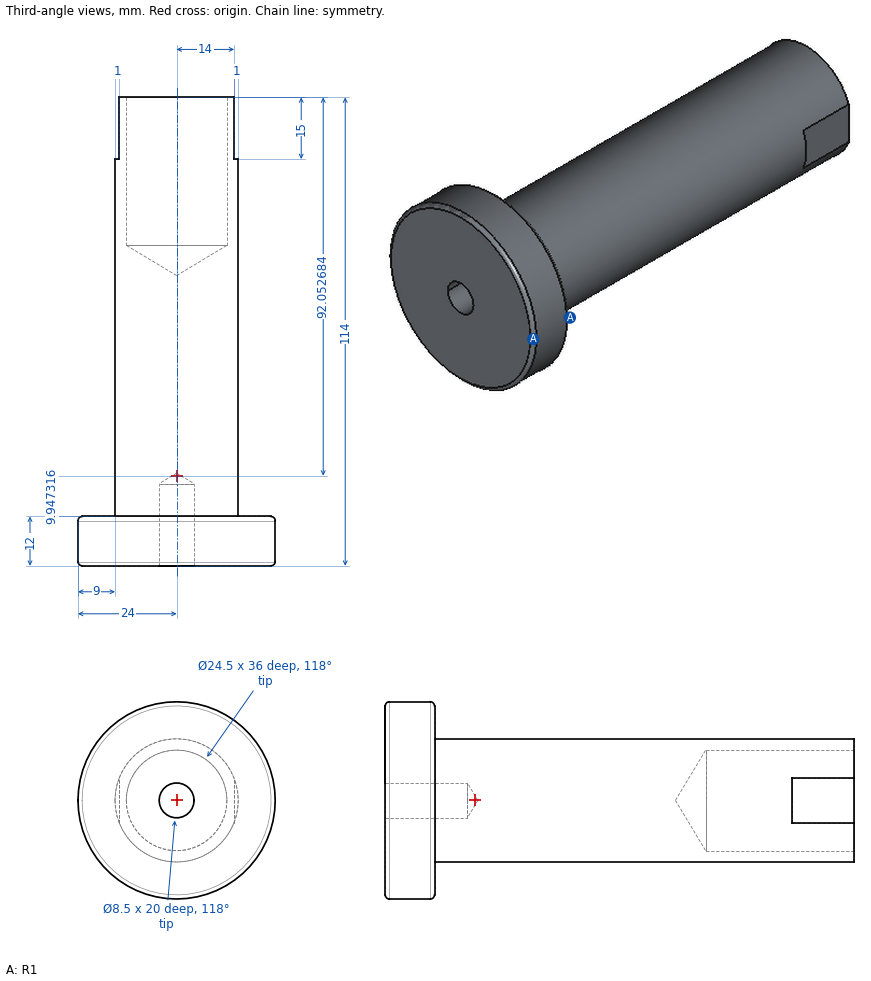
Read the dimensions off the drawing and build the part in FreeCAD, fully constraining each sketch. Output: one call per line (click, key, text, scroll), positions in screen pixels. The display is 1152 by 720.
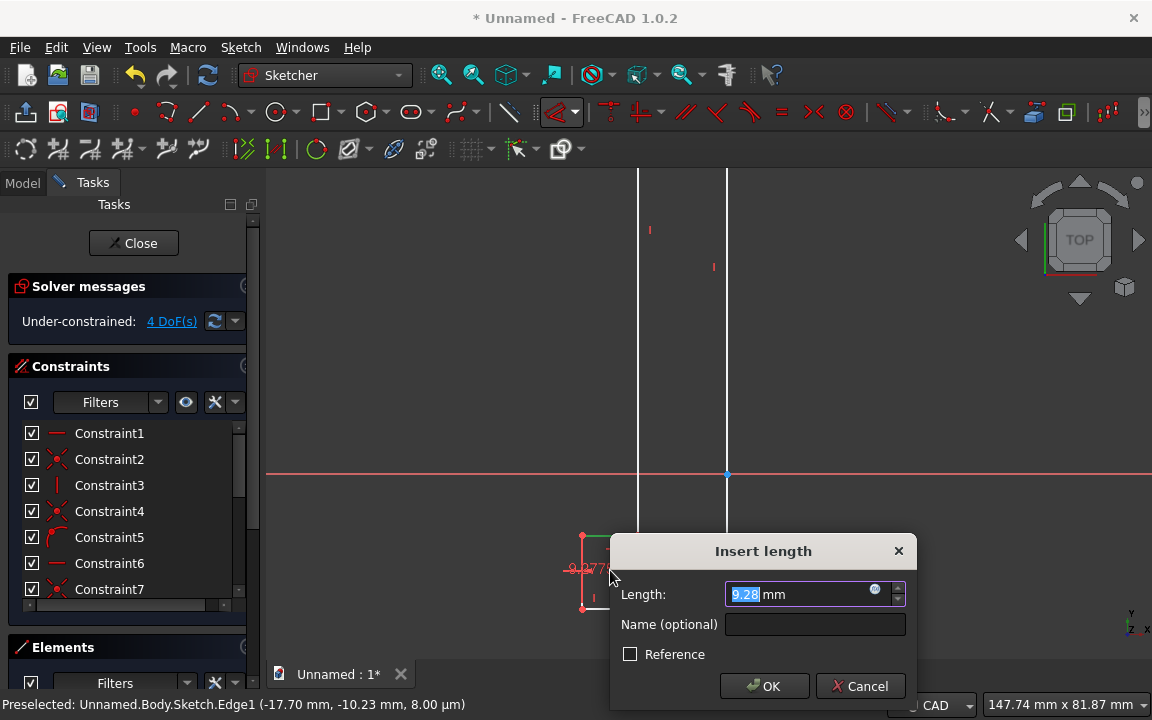
text(9)
key(Return)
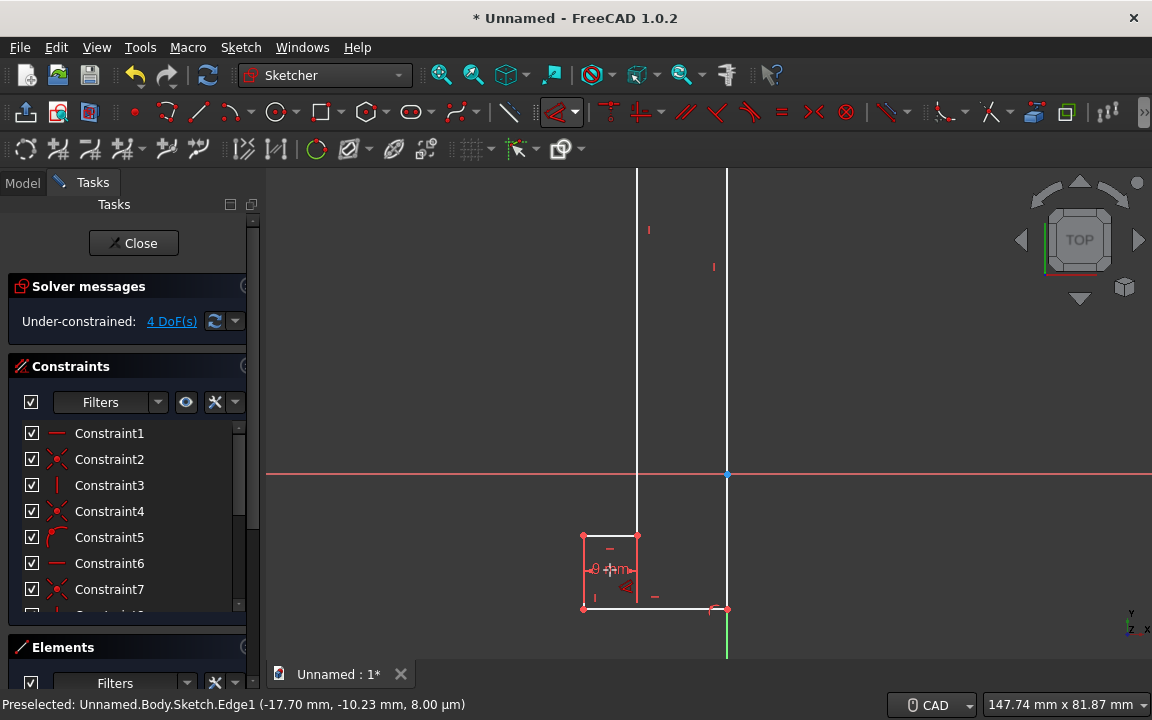
click(584, 558)
click(550, 547)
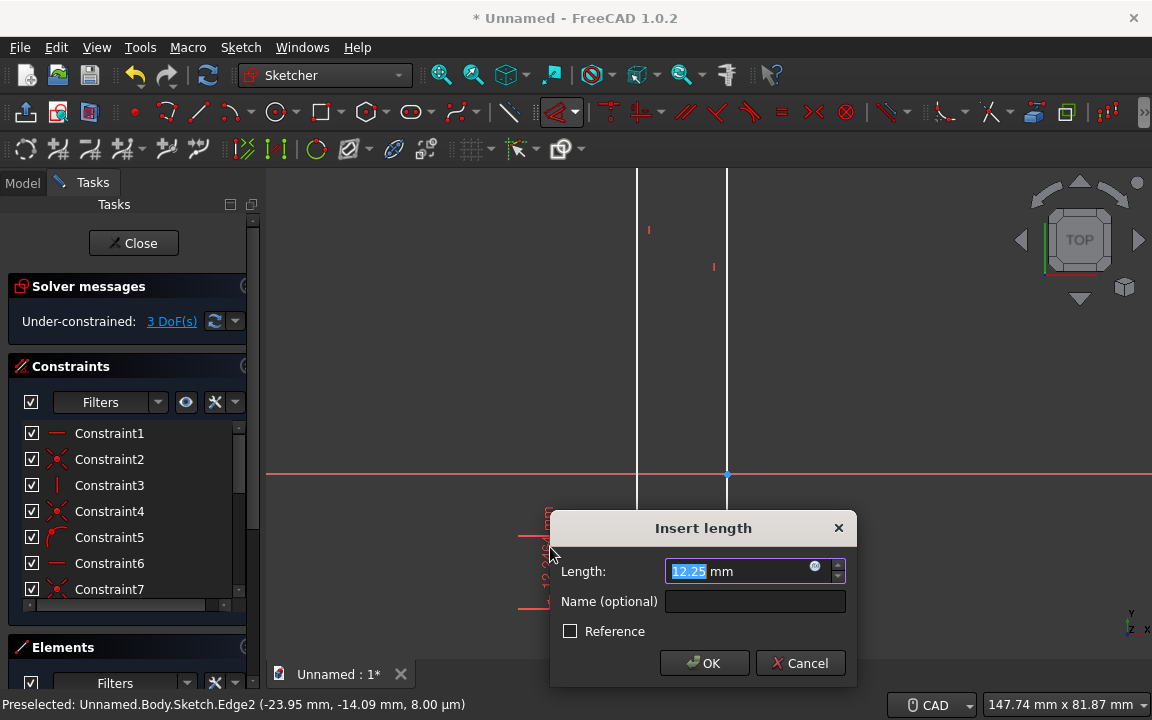
text(12)
key(Return)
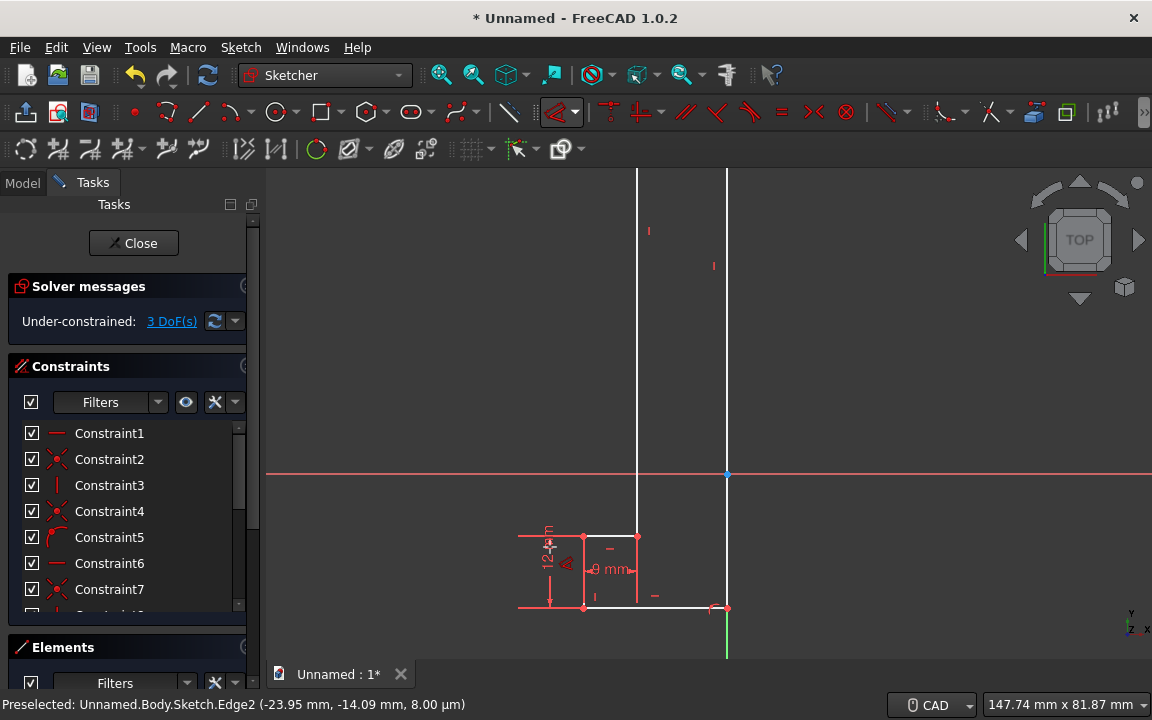
click(627, 608)
click(688, 574)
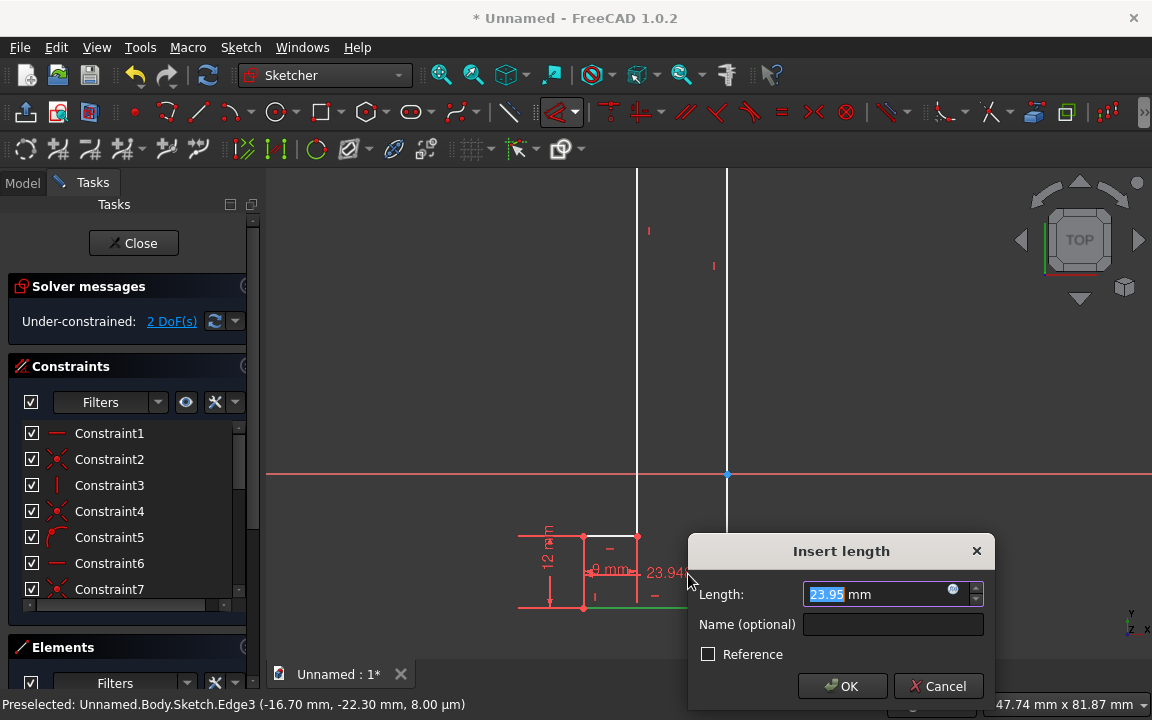
text(24)
key(Return)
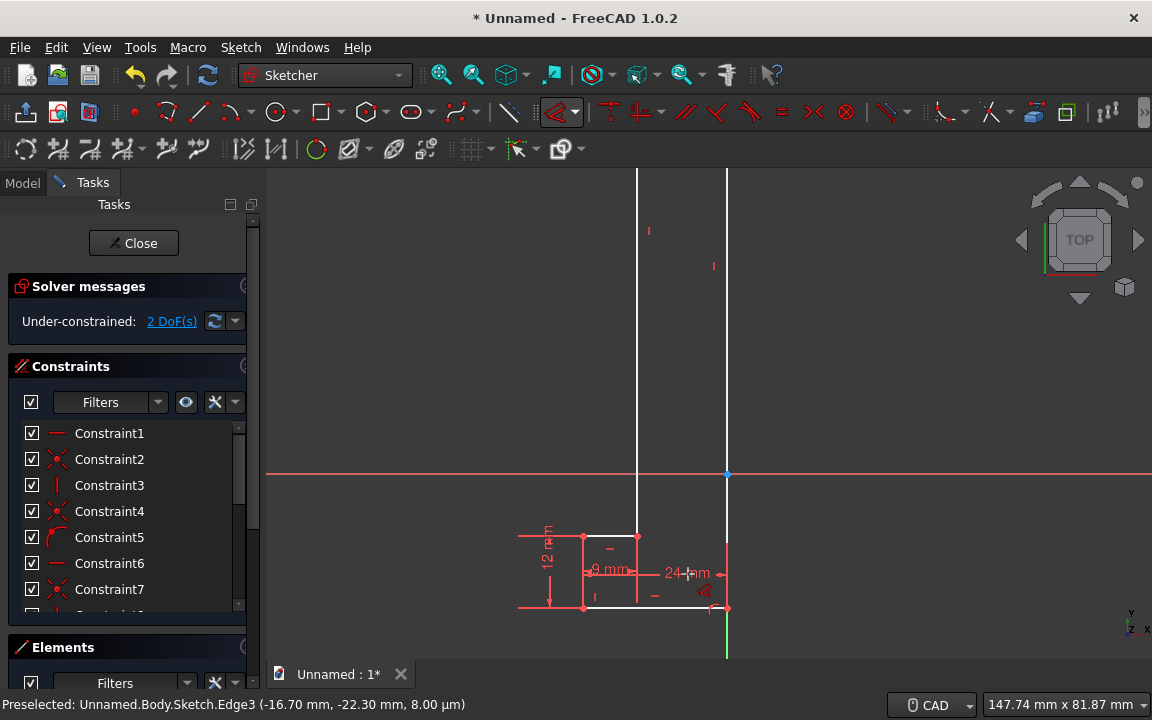
click(727, 403)
click(761, 402)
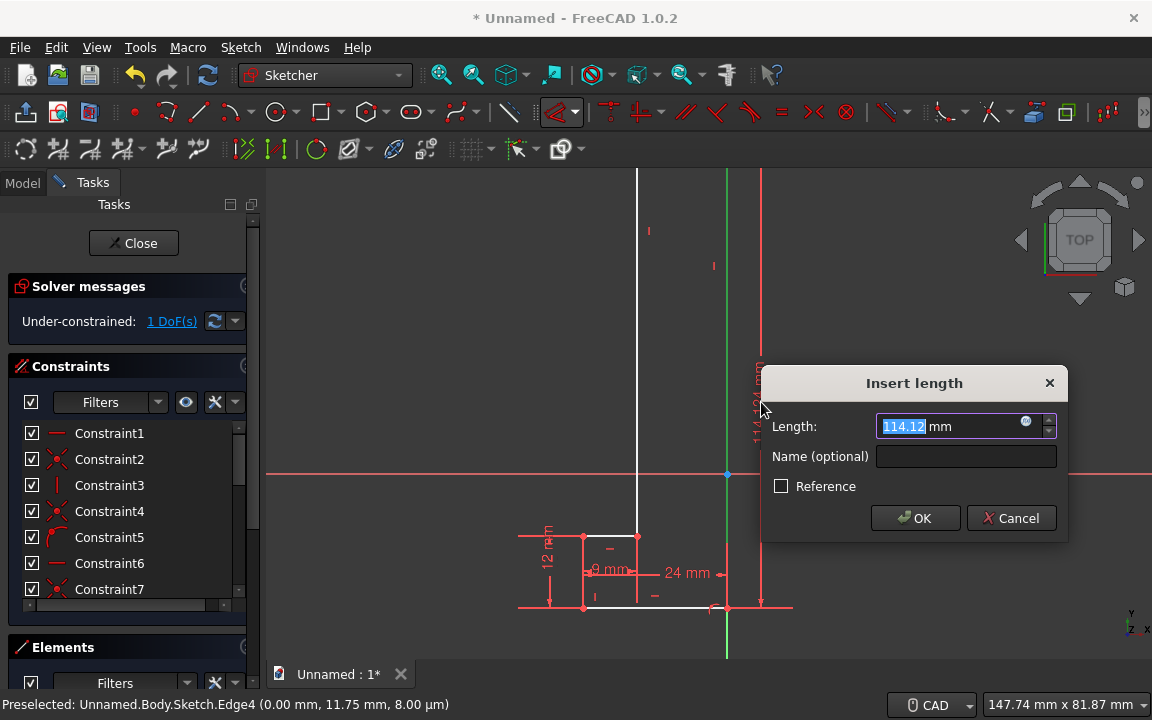
text(114)
key(Return)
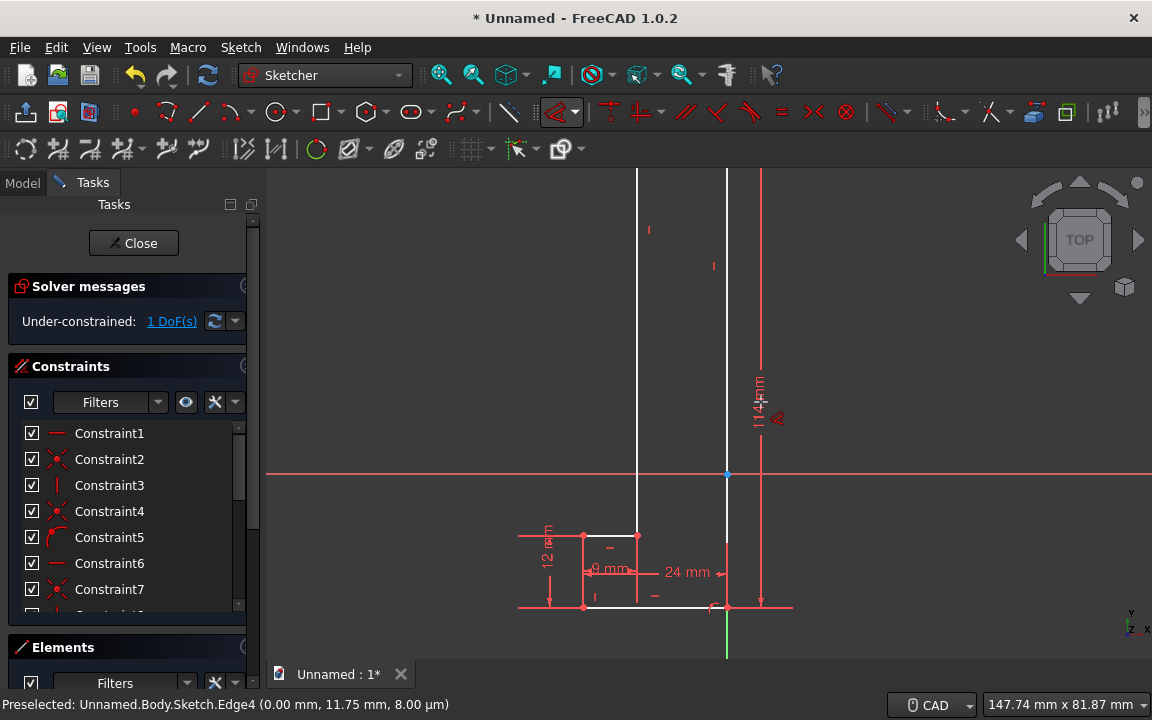
click(637, 536)
click(761, 505)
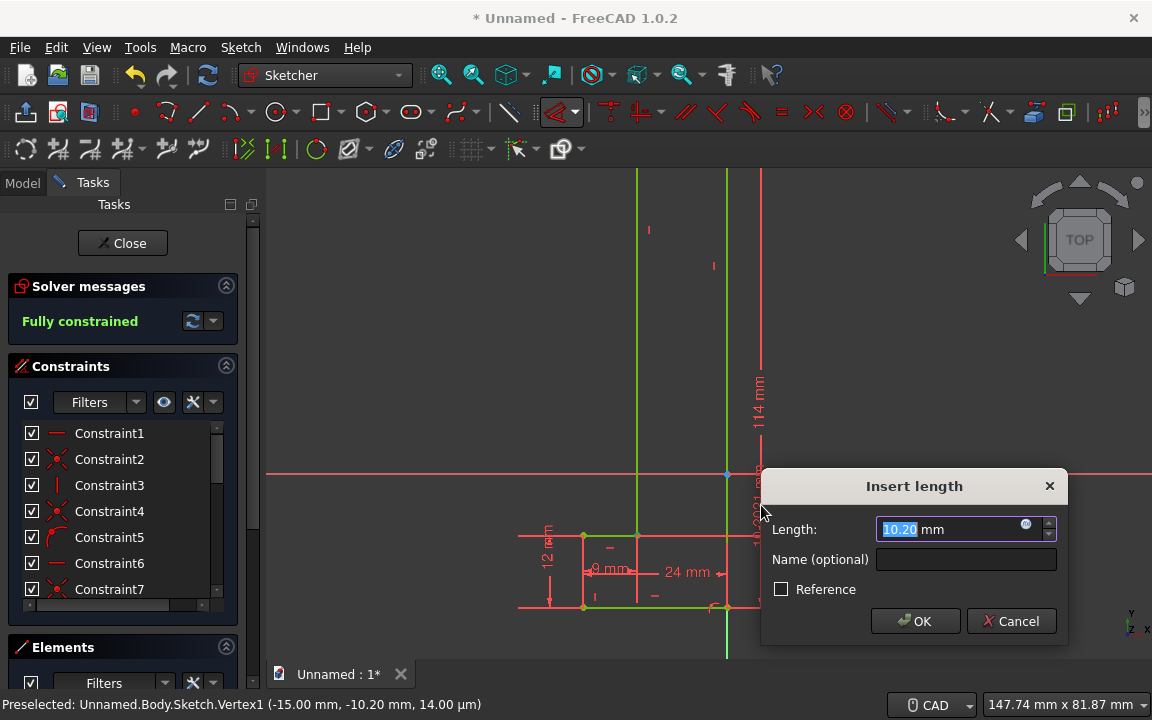
text(9.947316)
key(Return)
key(Escape)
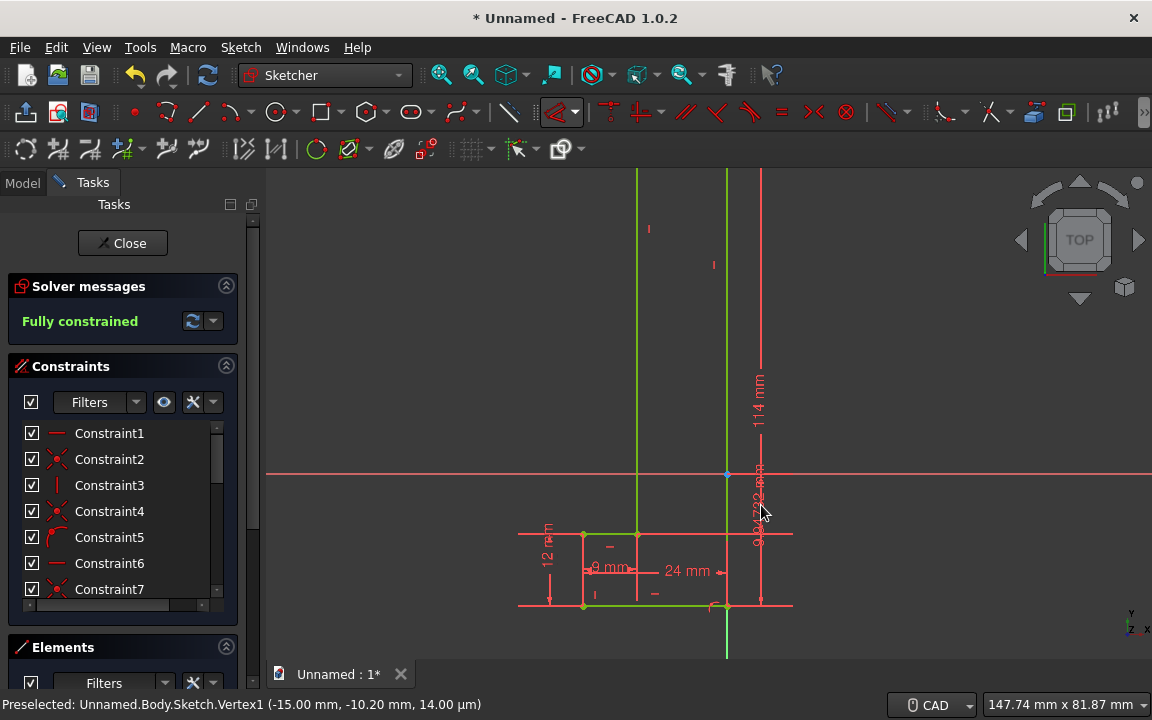
click(123, 243)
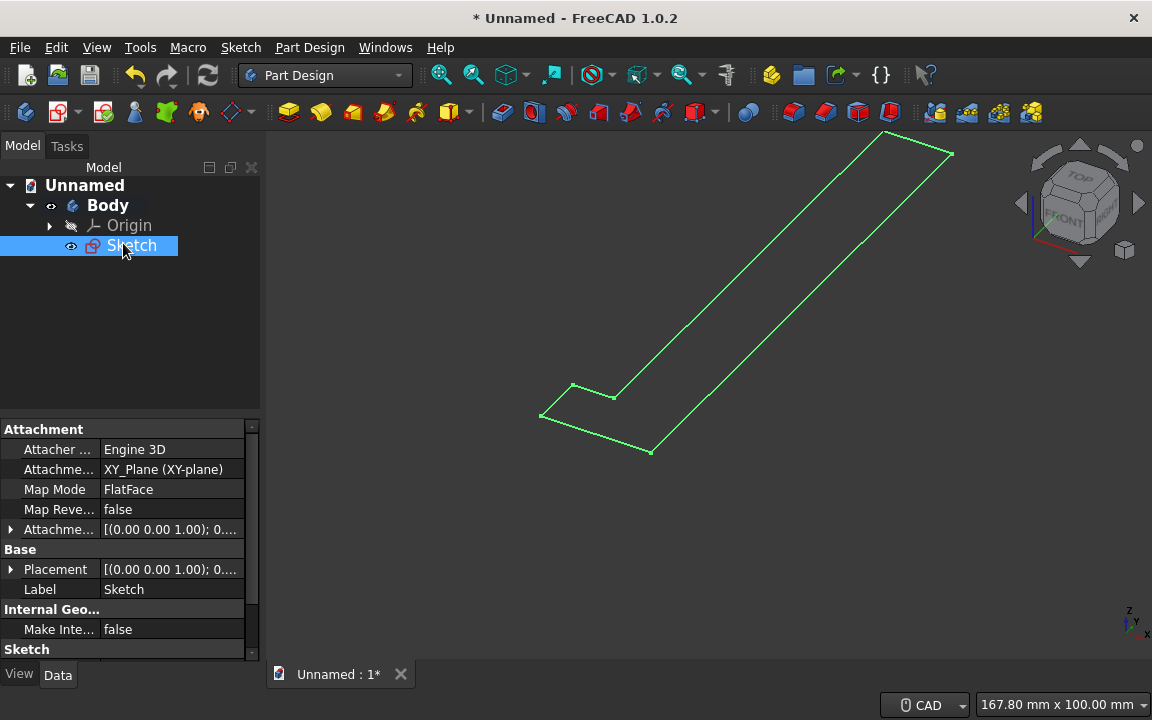
click(322, 112)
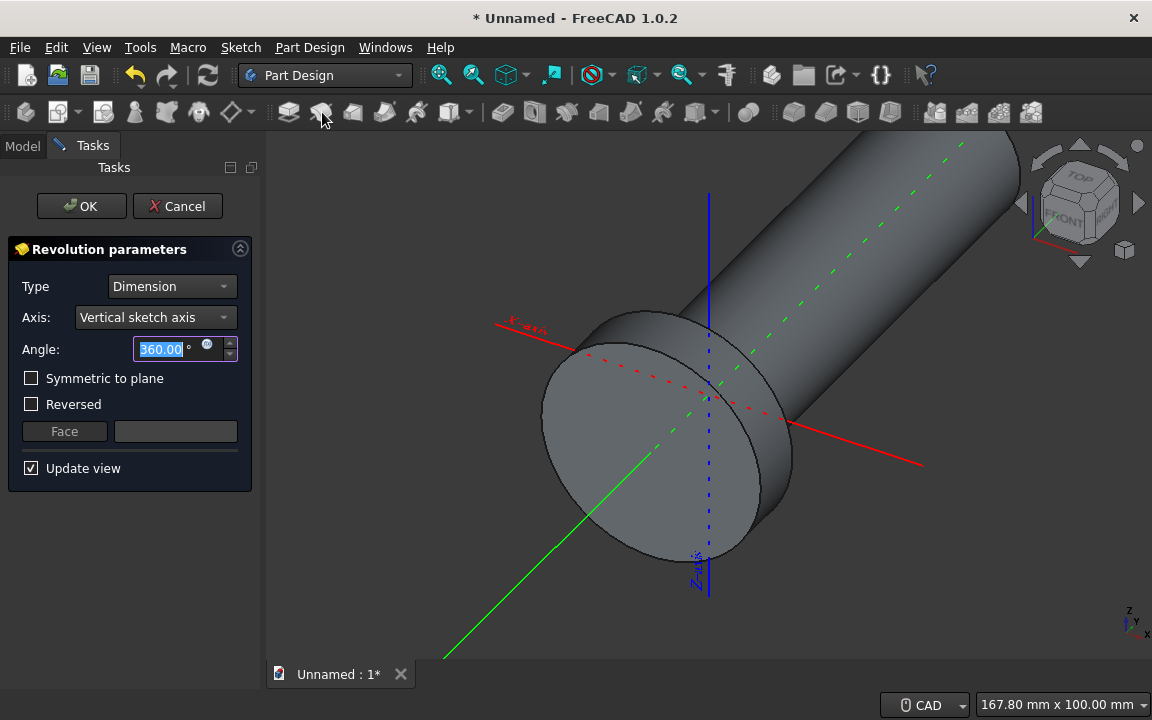
click(82, 206)